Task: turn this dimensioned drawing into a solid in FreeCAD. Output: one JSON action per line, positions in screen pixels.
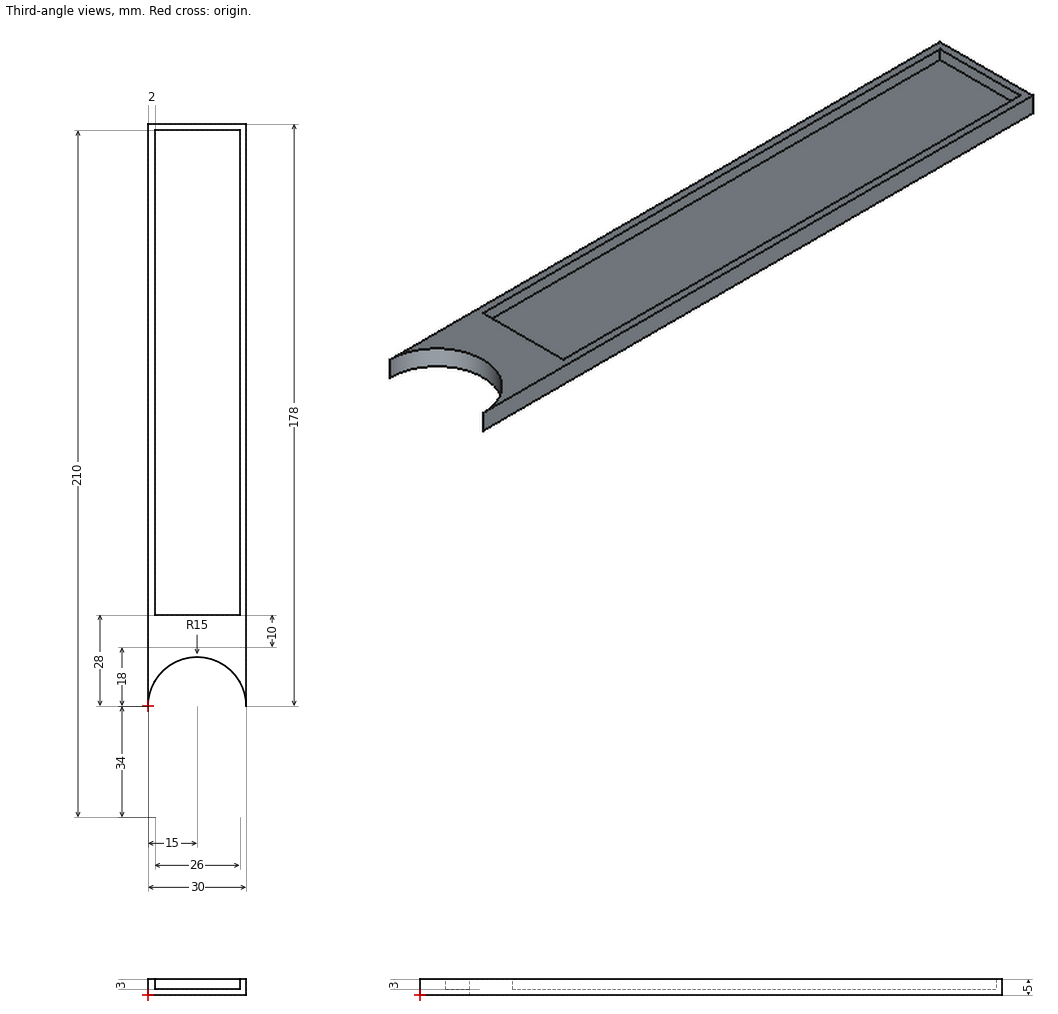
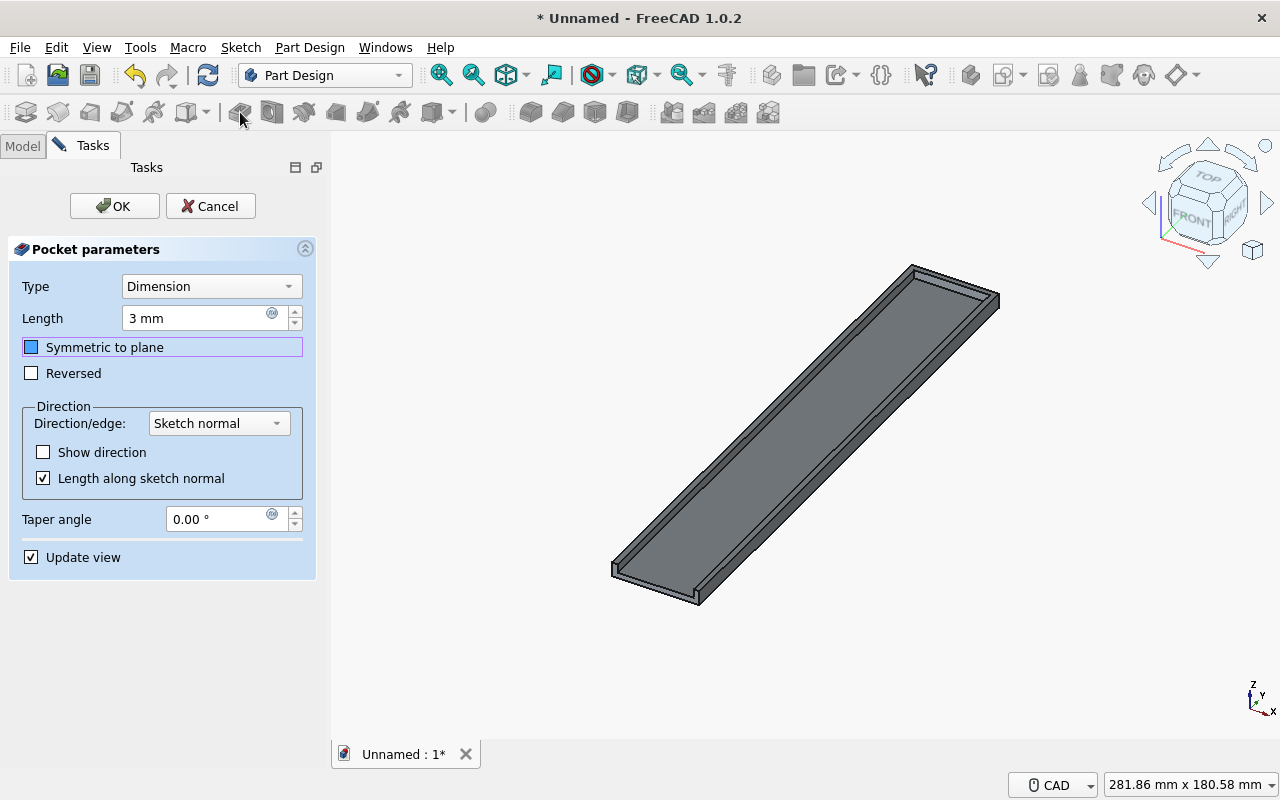
{"action": "left_click", "coordinate": [115, 206]}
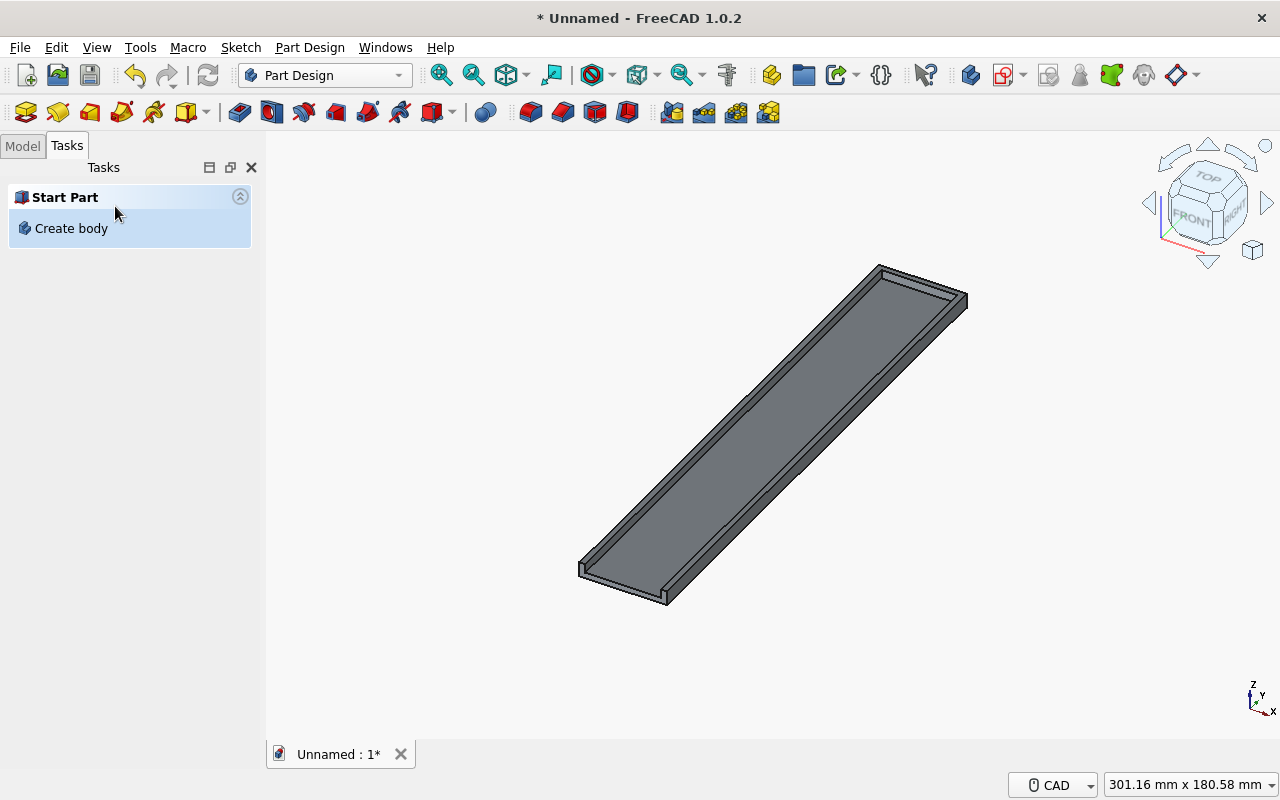
{"action": "left_click", "coordinate": [856, 353]}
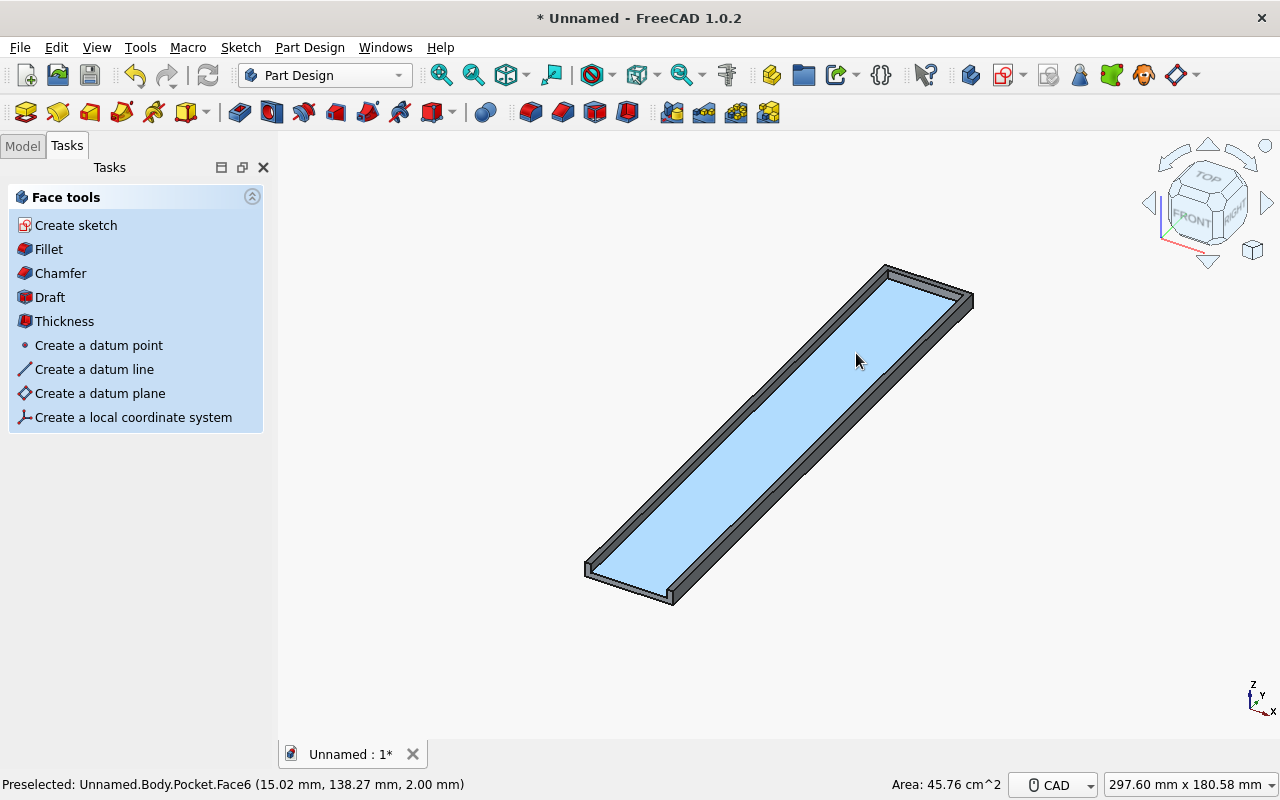
{"action": "left_click", "coordinate": [1004, 76]}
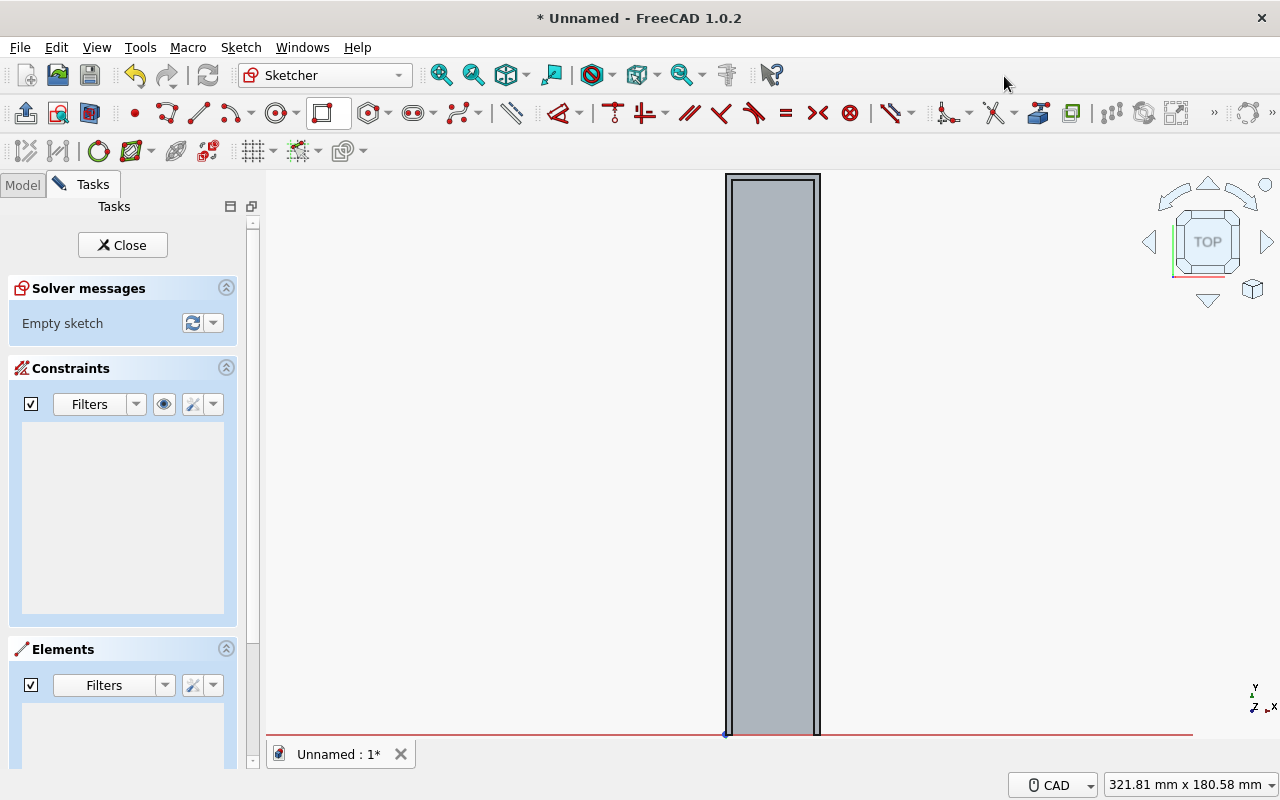
{"action": "scroll", "coordinate": [704, 454], "scroll_direction": "down", "scroll_amount": 5}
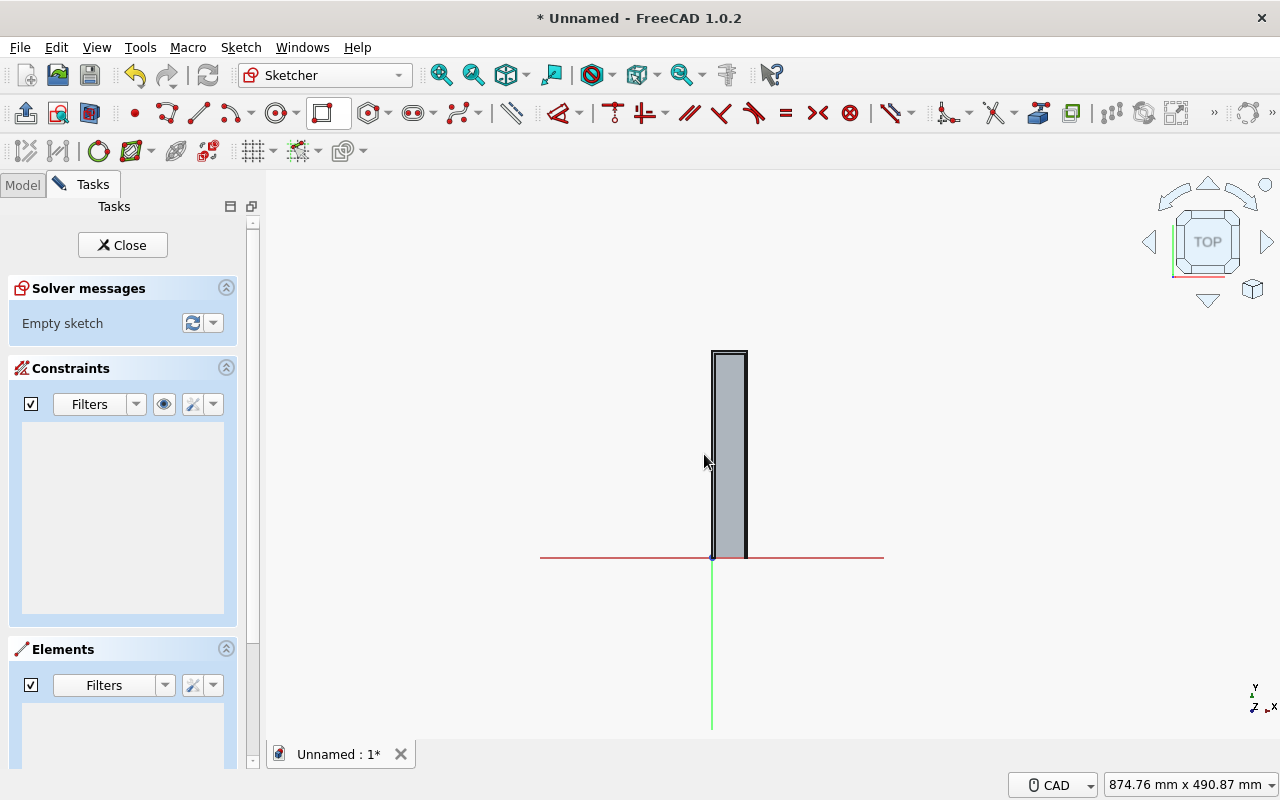
{"action": "scroll", "coordinate": [731, 550], "scroll_direction": "up", "scroll_amount": 12}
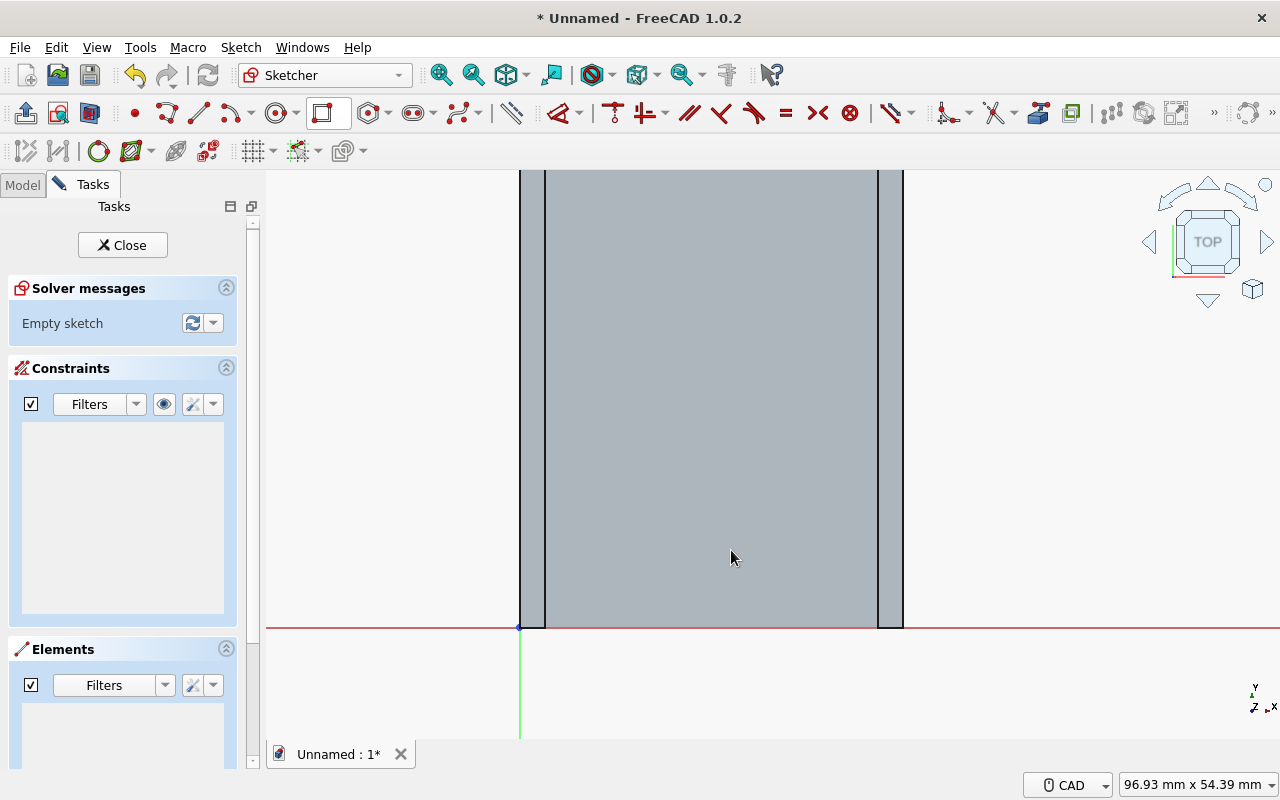
{"action": "key", "text": "g r"}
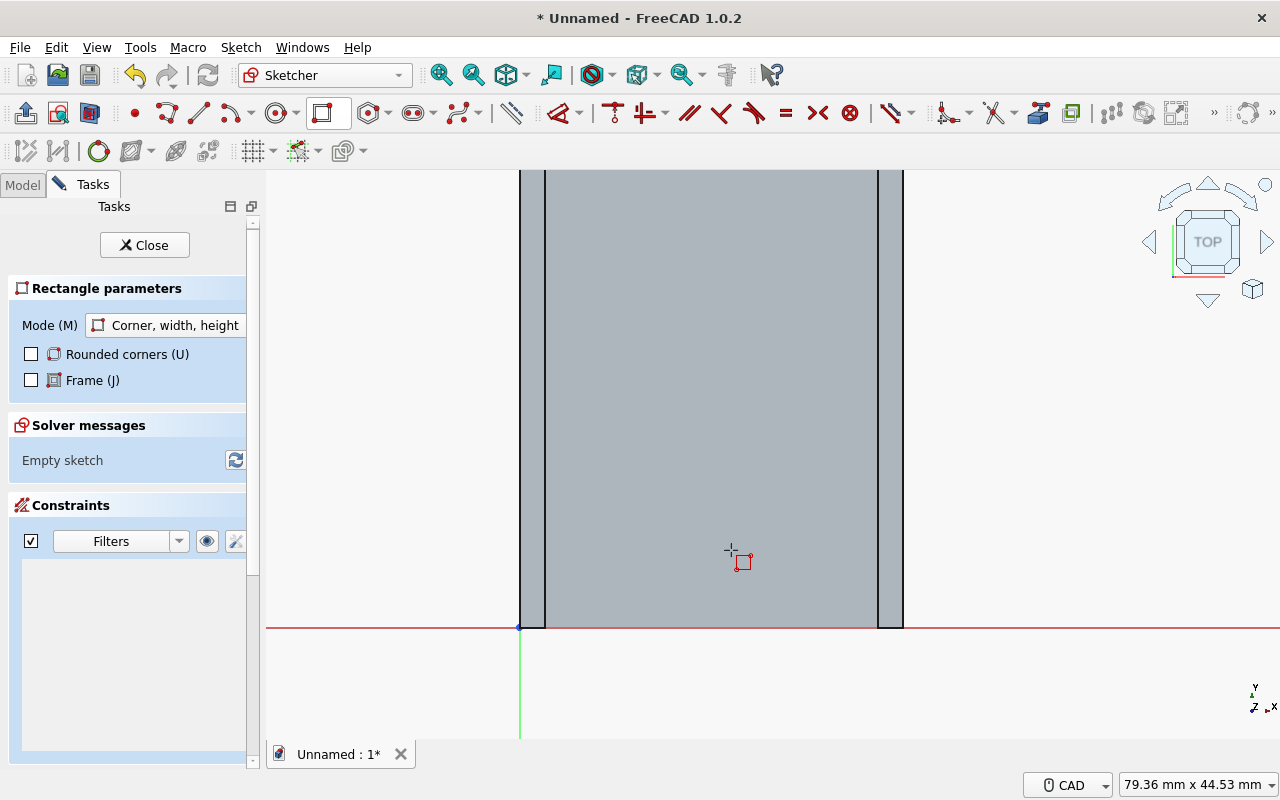
{"action": "left_click", "coordinate": [545, 270]}
{"action": "mouse_move", "coordinate": [878, 398]}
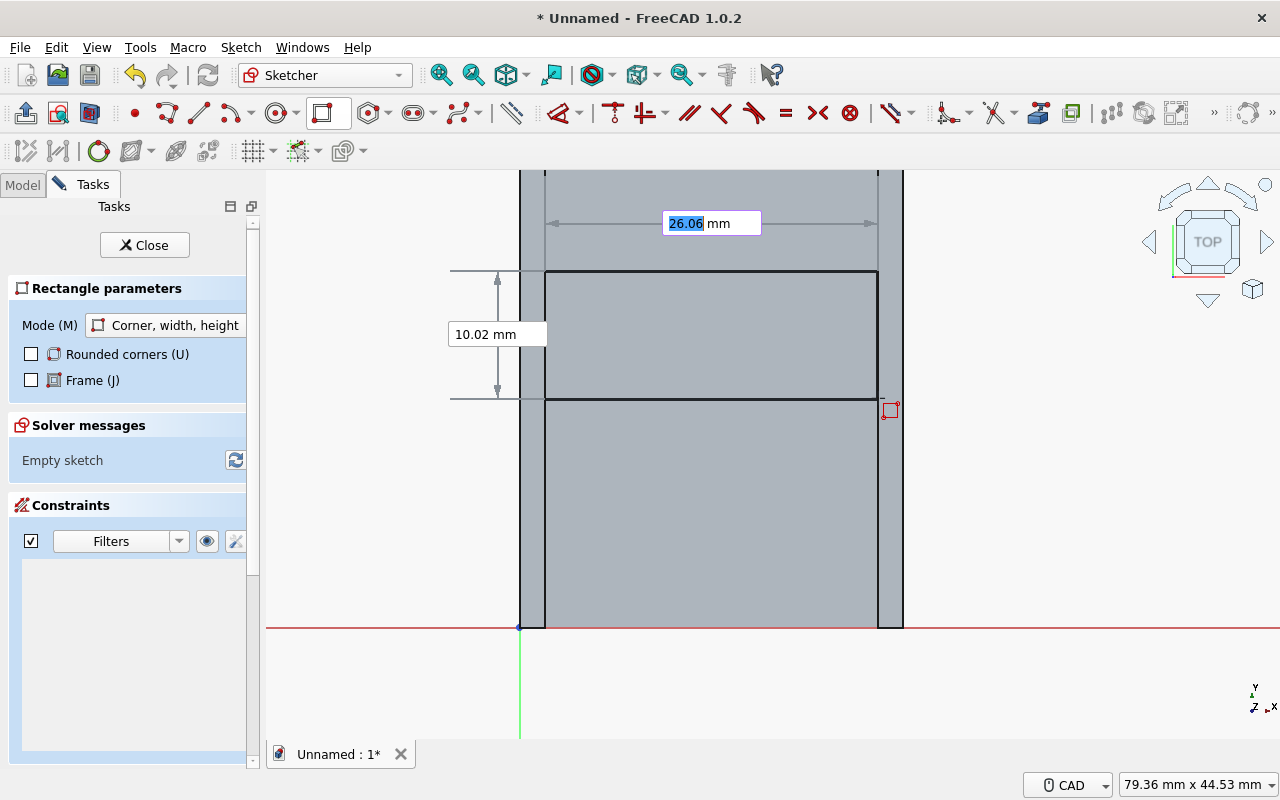
{"action": "type", "text": "26"}
{"action": "key", "text": "Tab"}
{"action": "type", "text": "10"}
{"action": "key", "text": "Return"}
{"action": "key", "text": "Escape"}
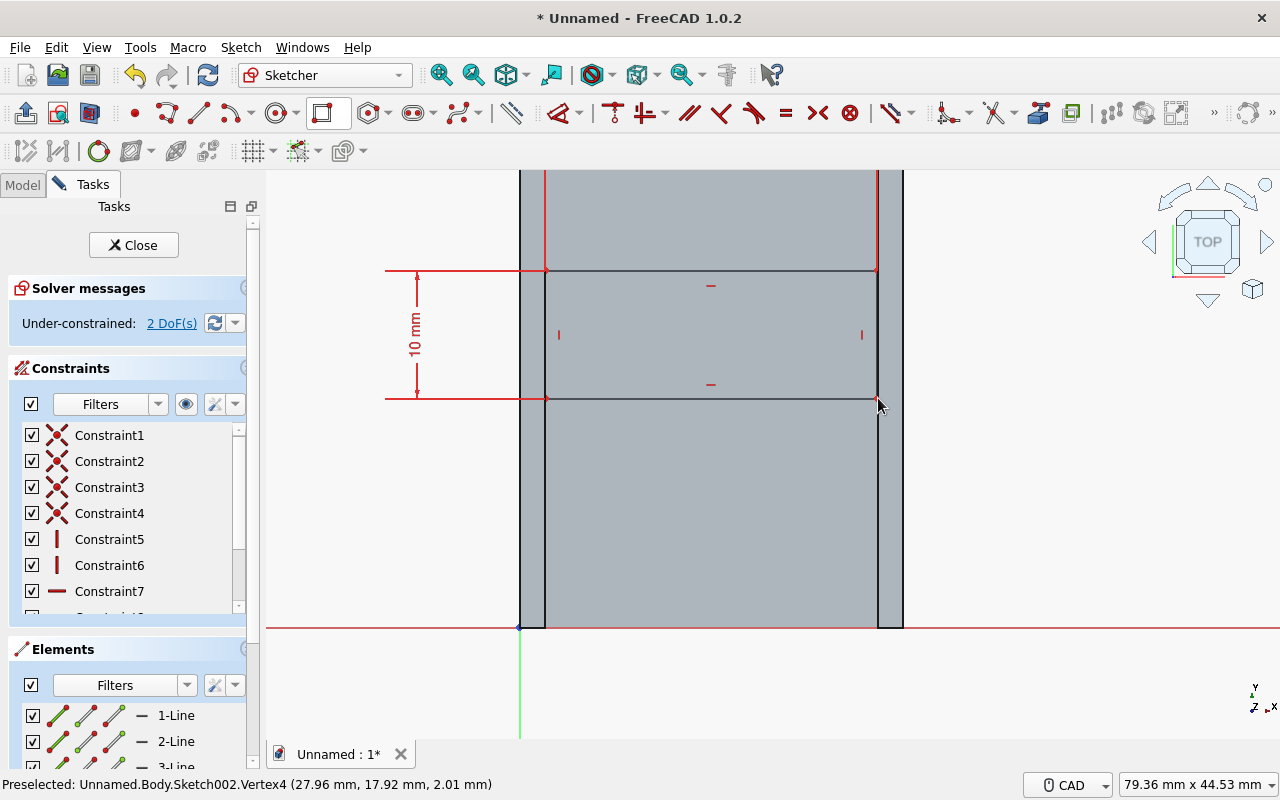
{"action": "scroll", "coordinate": [545, 271], "scroll_direction": "up", "scroll_amount": 3}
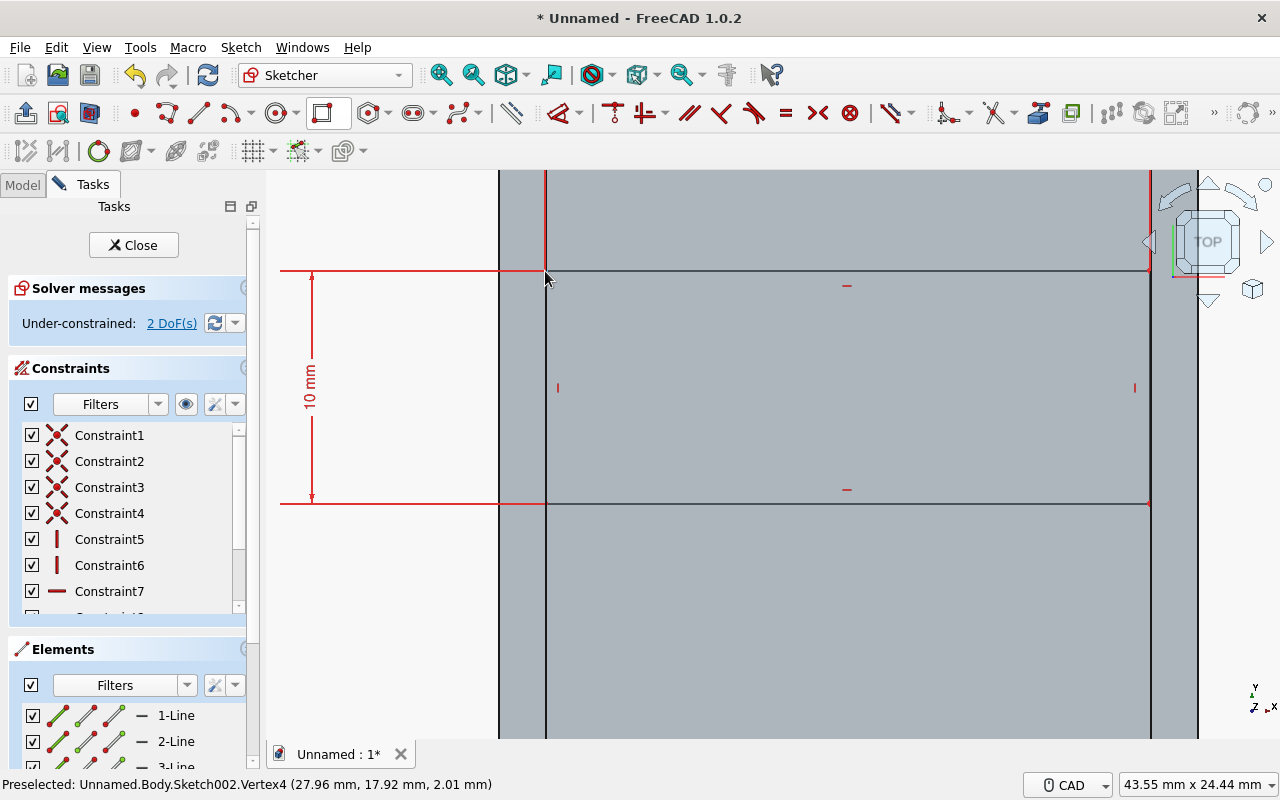
{"action": "left_click", "coordinate": [545, 271]}